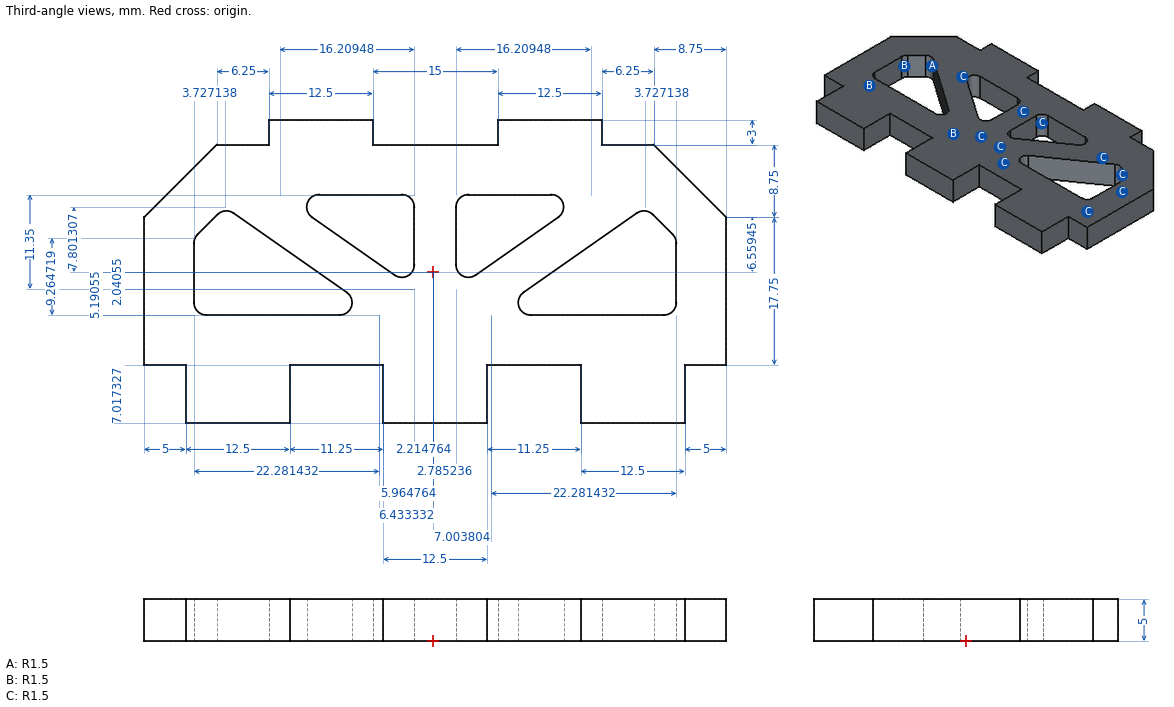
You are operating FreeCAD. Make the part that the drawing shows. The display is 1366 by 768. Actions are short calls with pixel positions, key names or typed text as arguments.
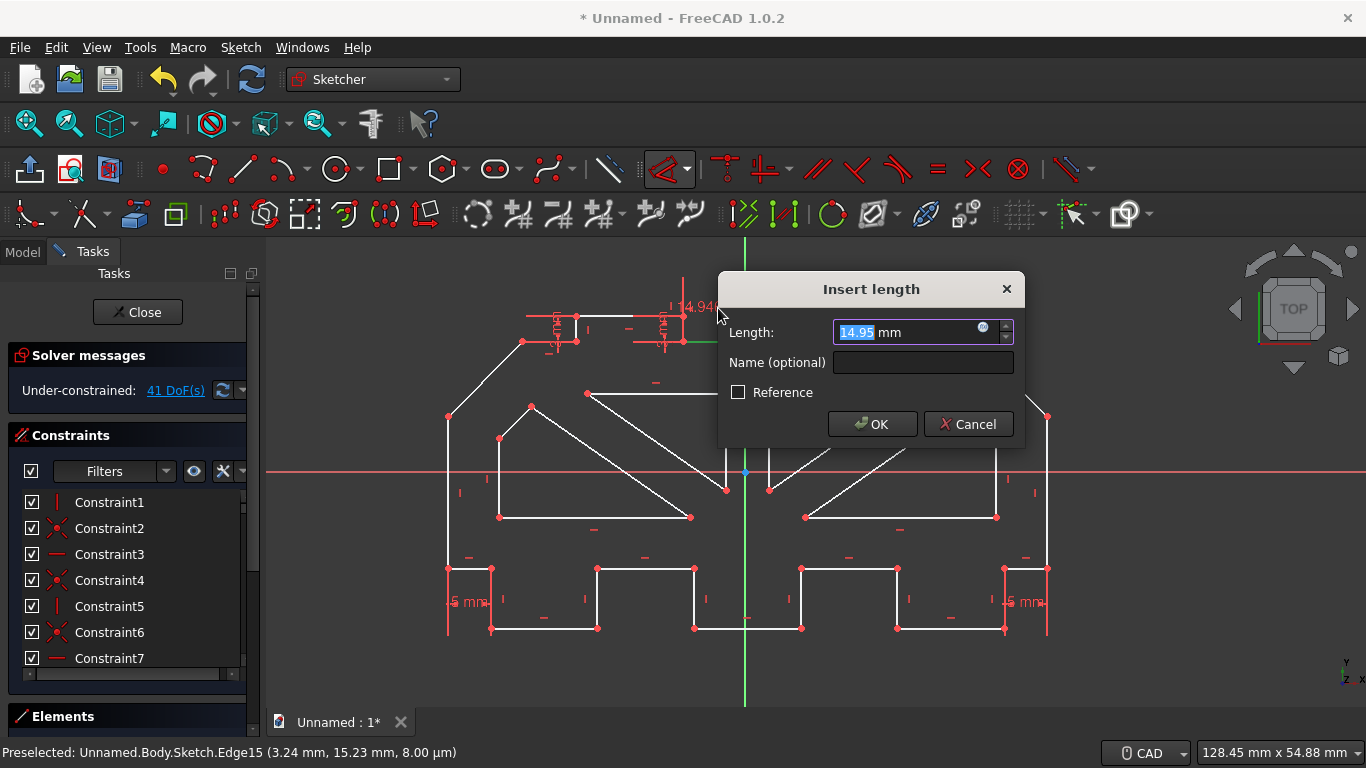
text(15)
key(Return)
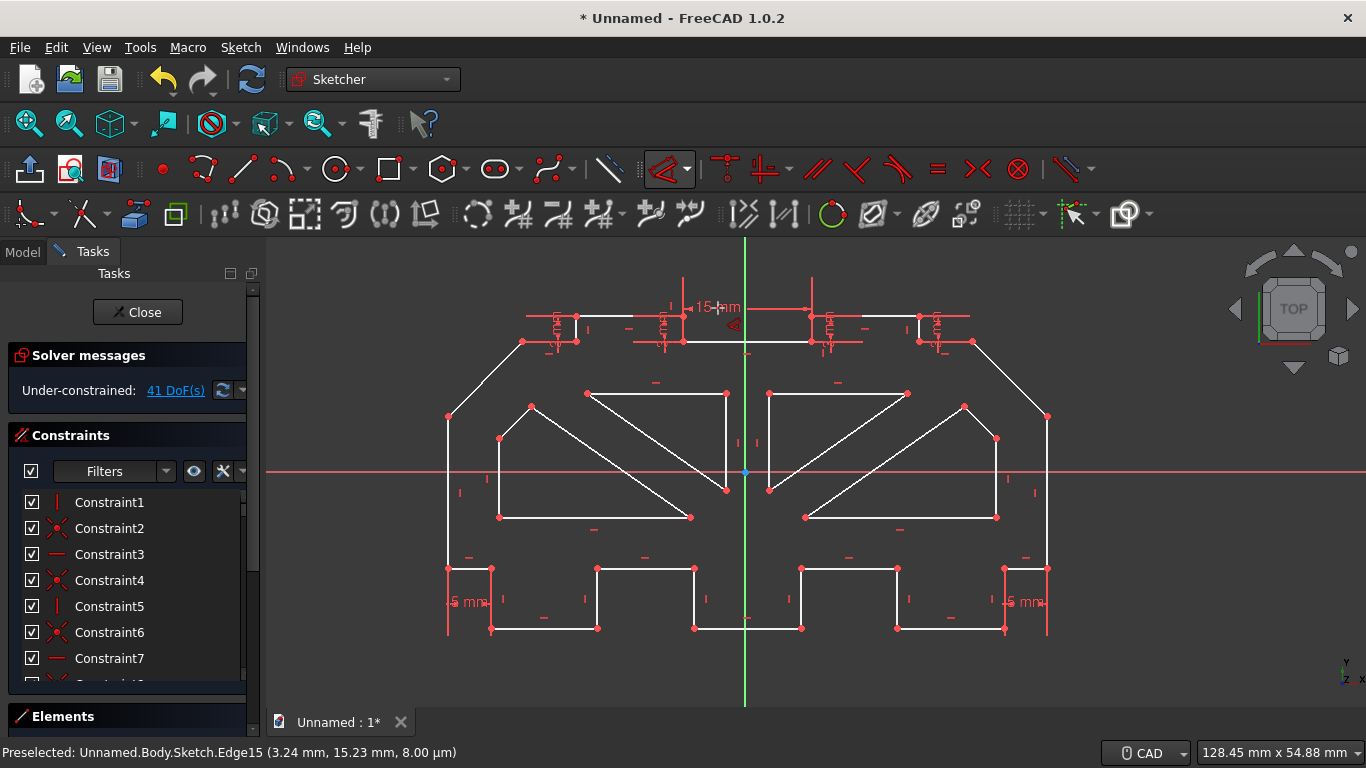
click(727, 629)
click(723, 663)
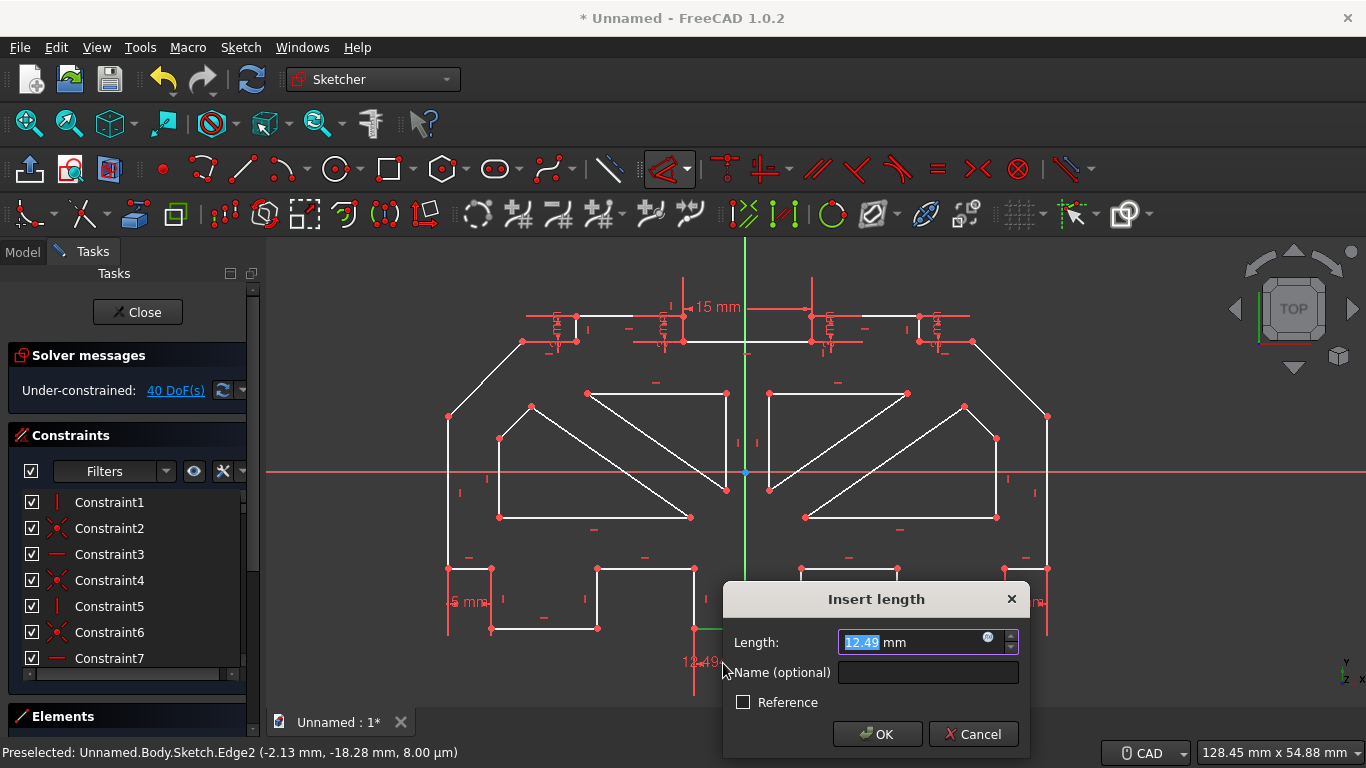
text(12.5)
key(Return)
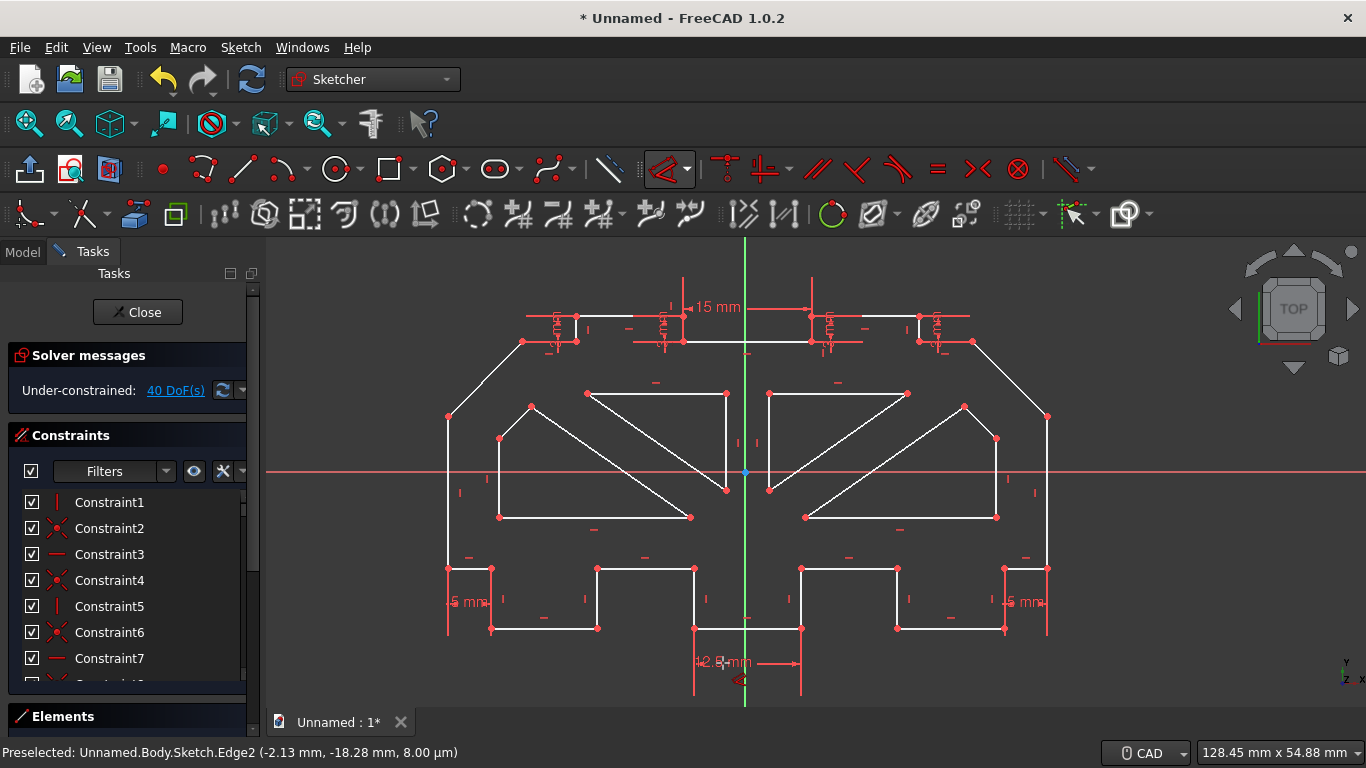
click(930, 629)
click(951, 663)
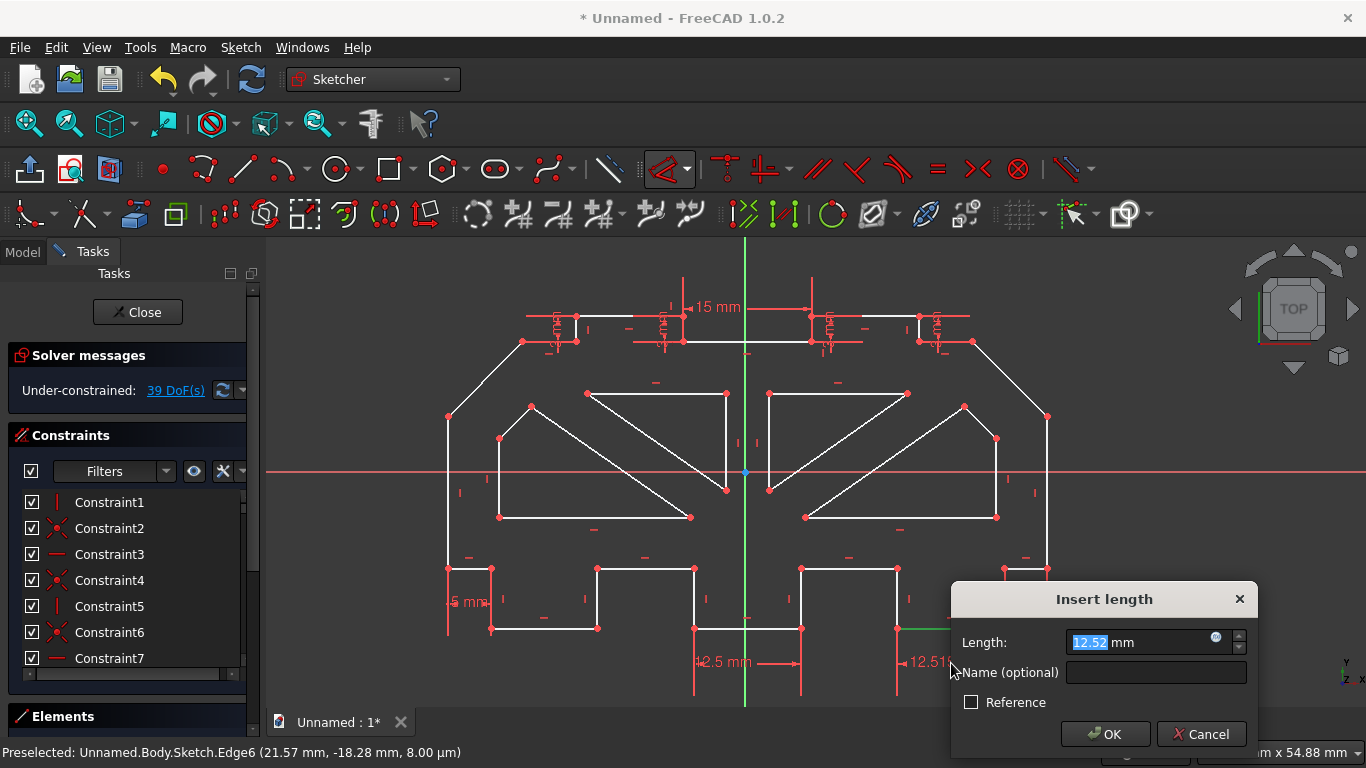
text(12.5)
key(Return)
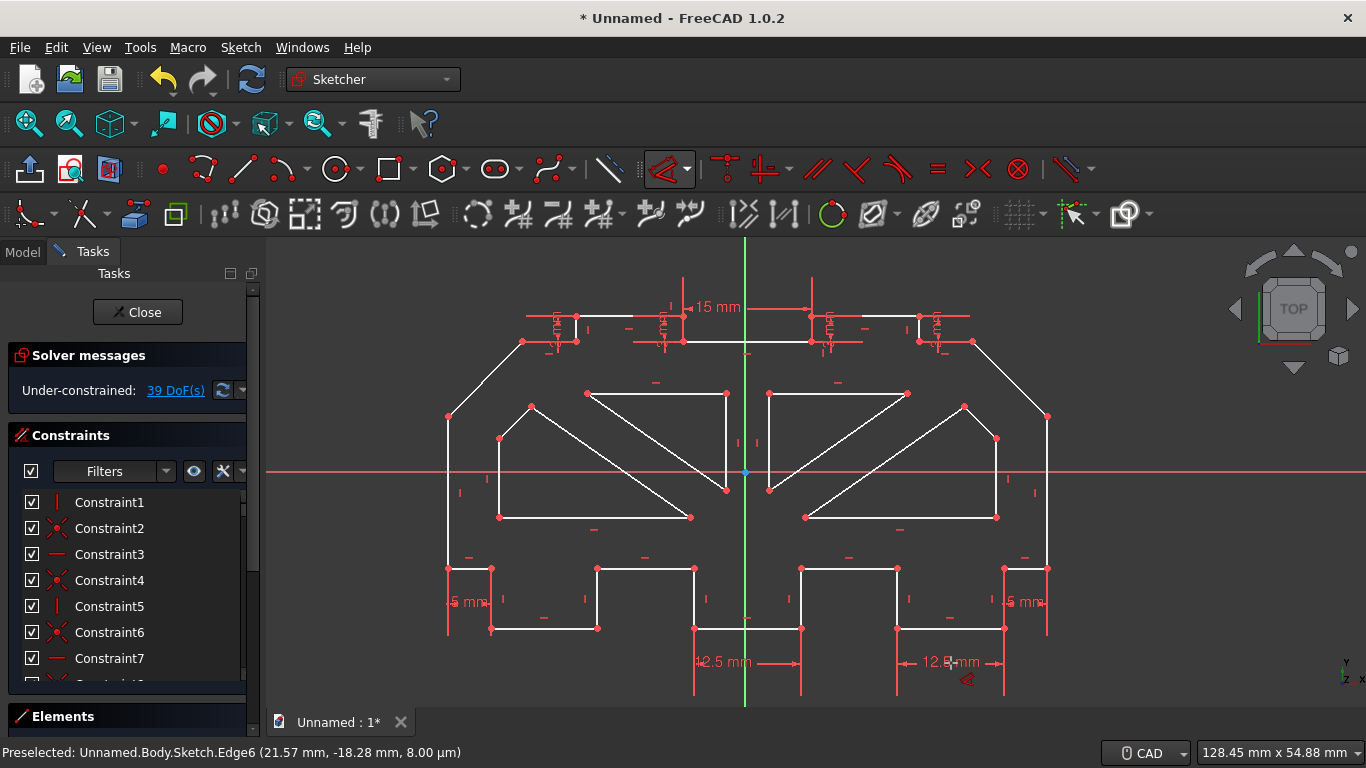
click(957, 342)
click(946, 308)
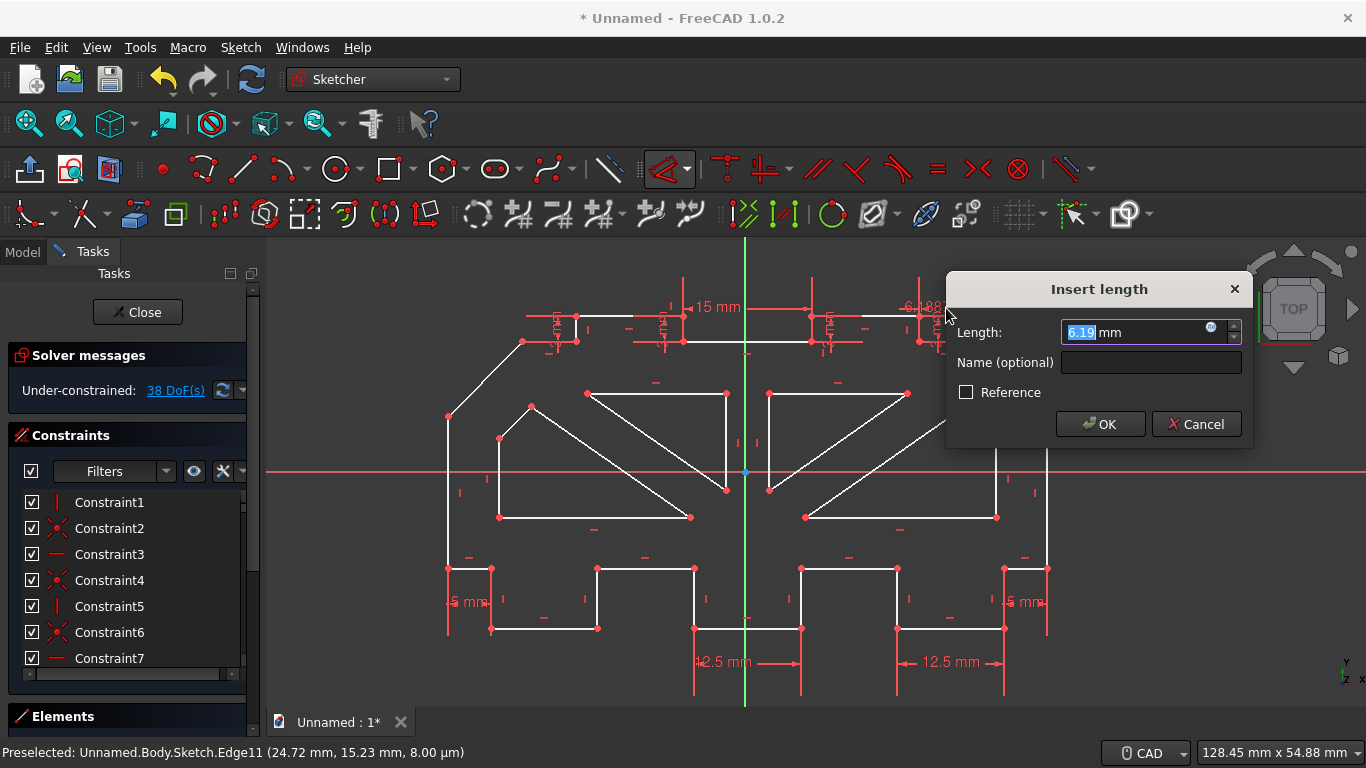
text(6.25)
key(Return)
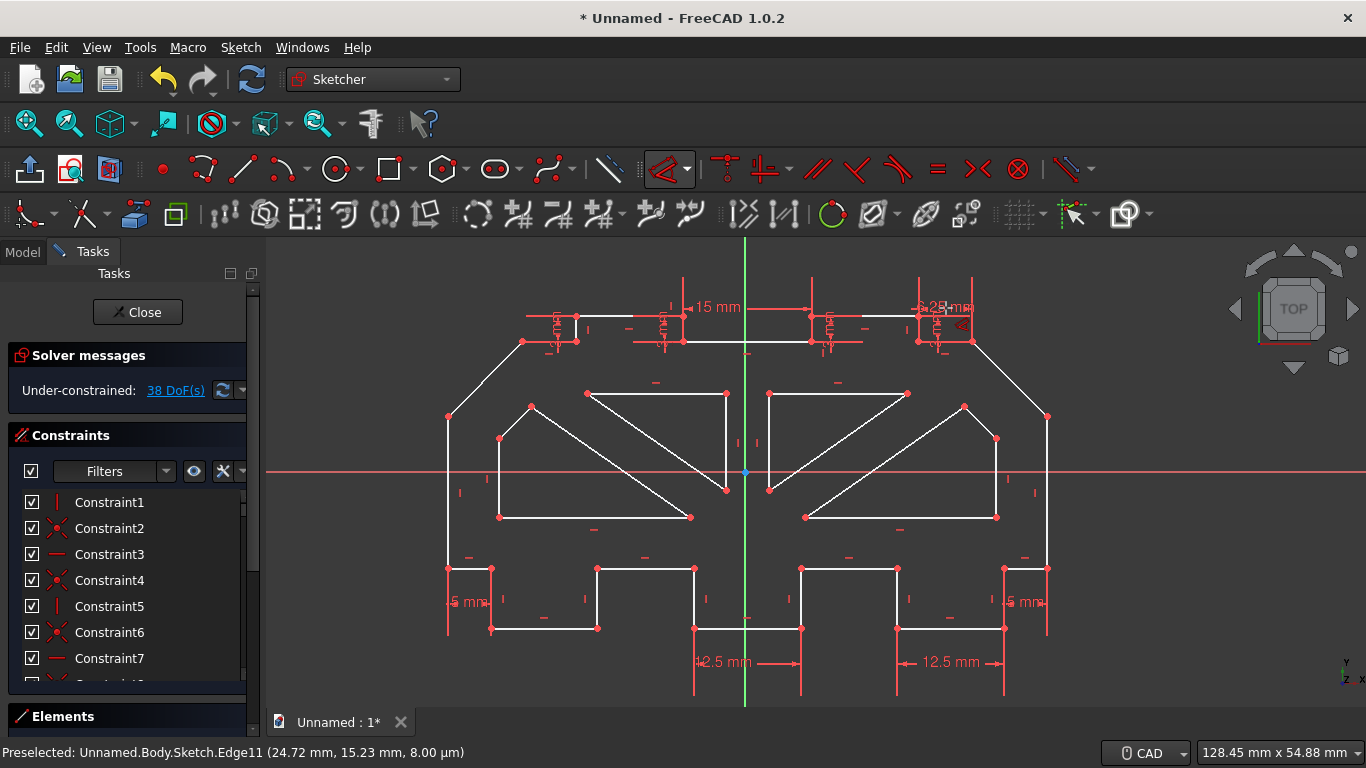
click(887, 316)
click(865, 282)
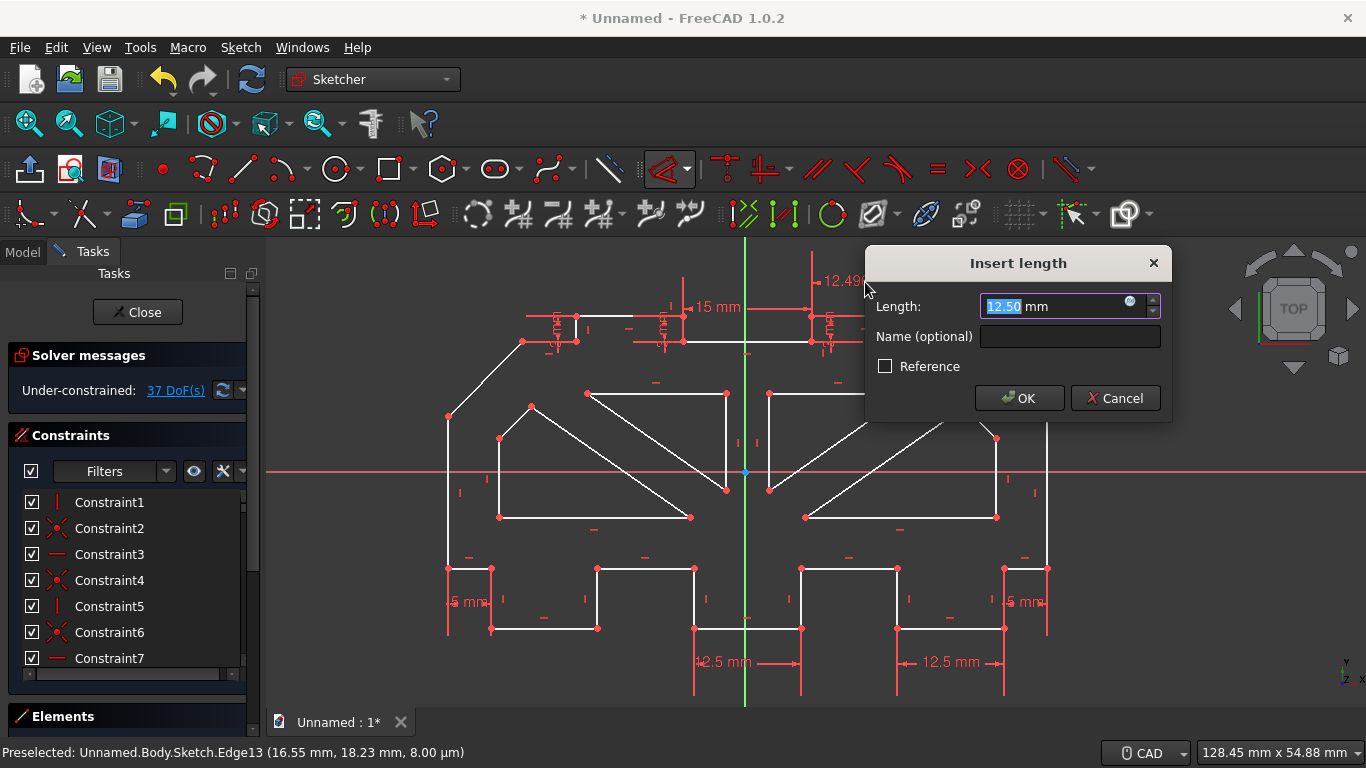
text(12.5)
key(Return)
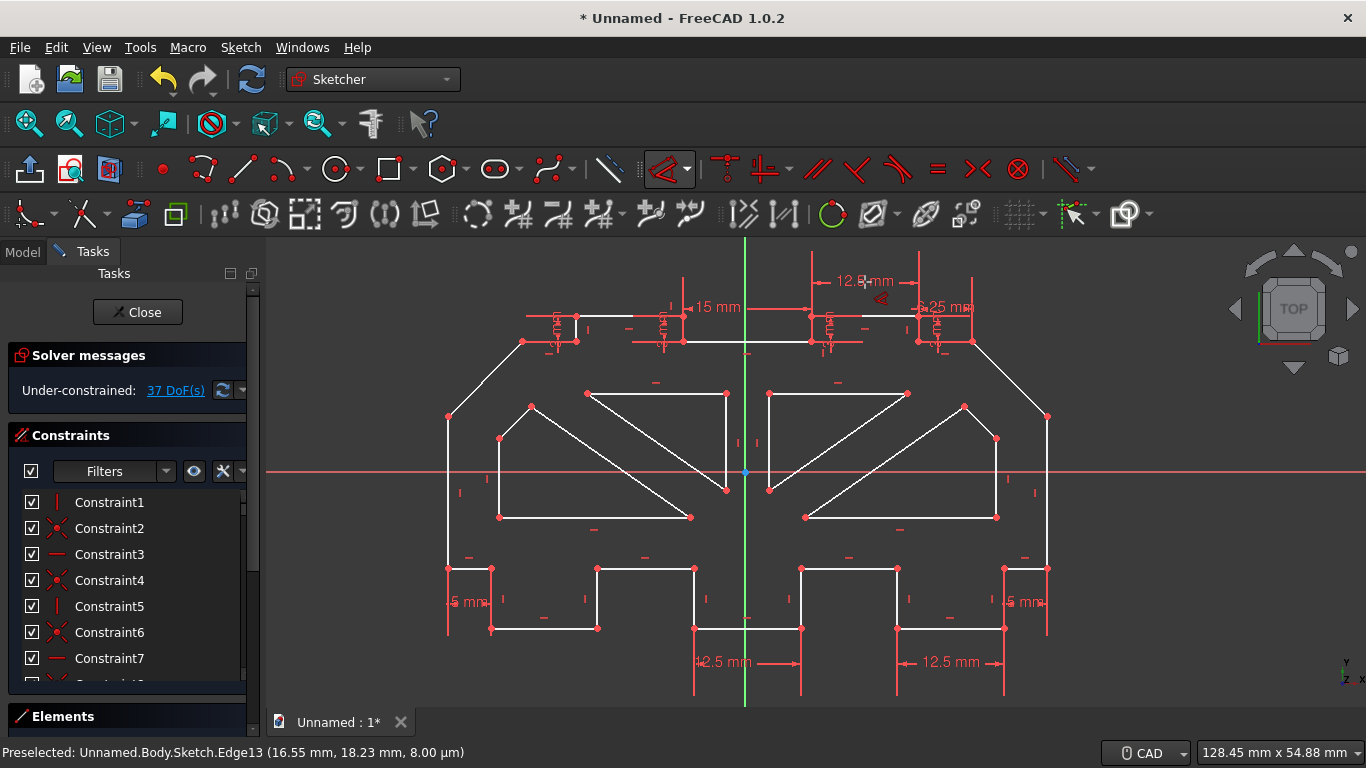
click(651, 316)
click(630, 282)